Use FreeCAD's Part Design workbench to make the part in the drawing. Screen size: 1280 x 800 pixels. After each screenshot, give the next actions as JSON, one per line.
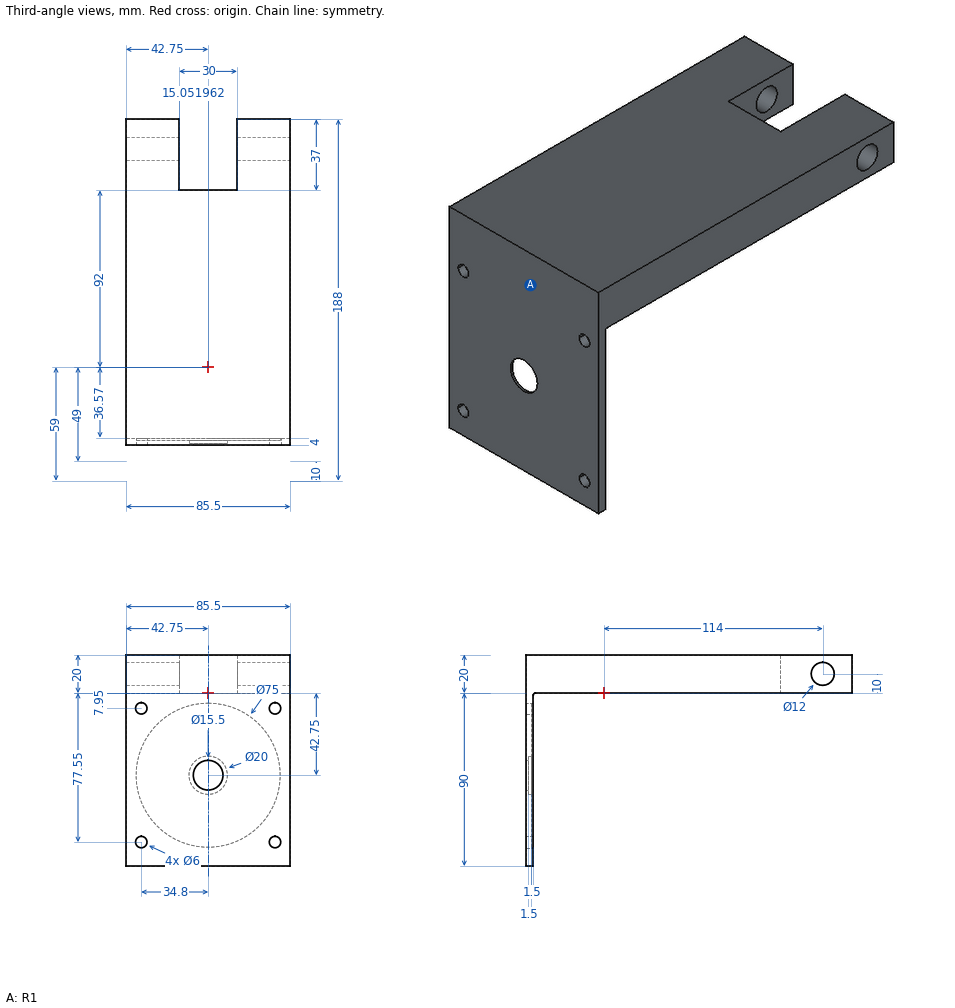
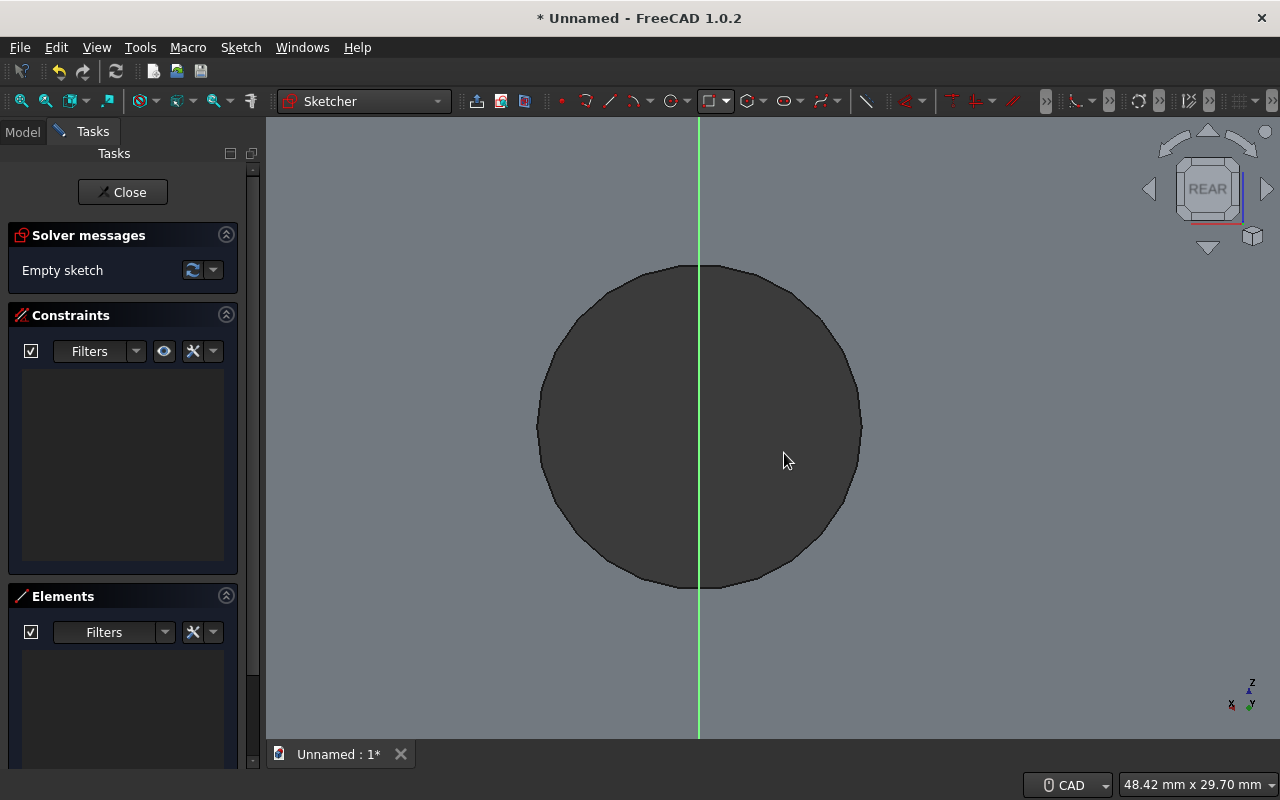
{"action": "key", "text": "g c"}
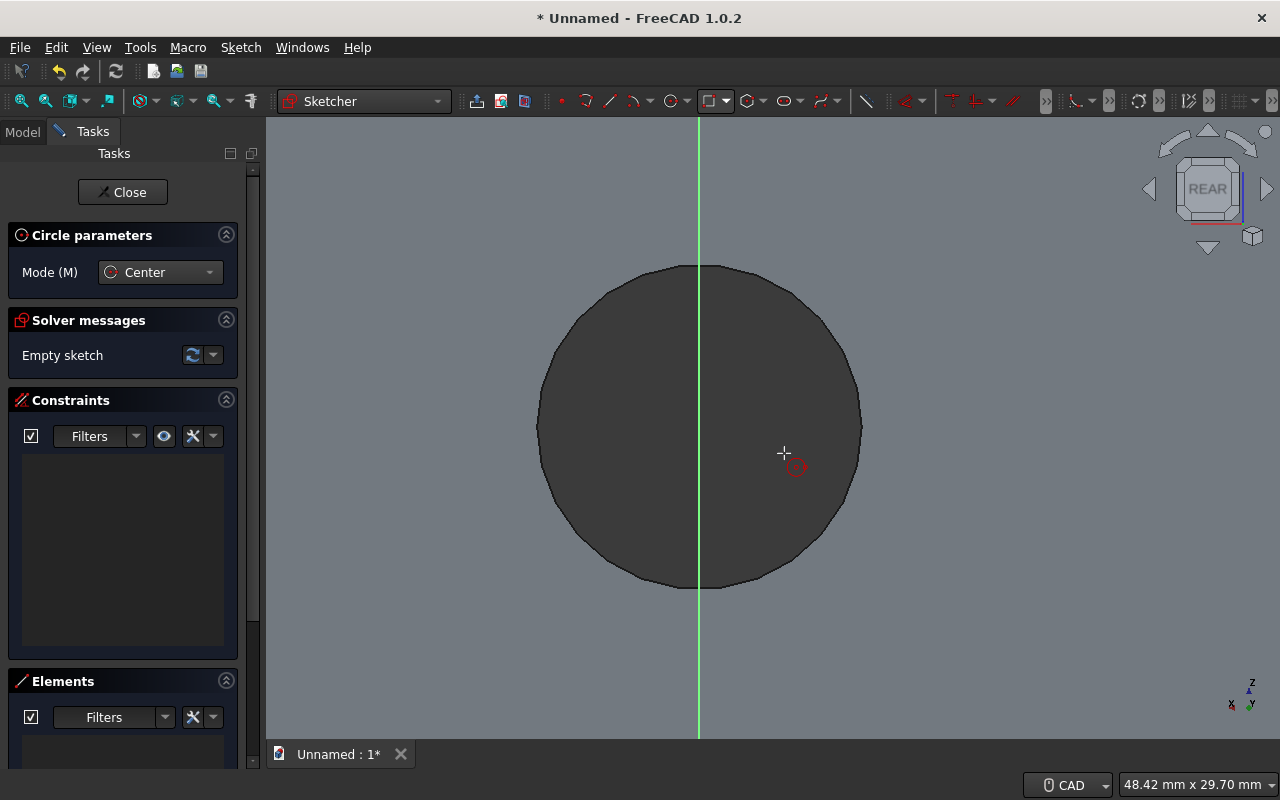
{"action": "left_click", "coordinate": [699, 427]}
{"action": "mouse_move", "coordinate": [848, 279]}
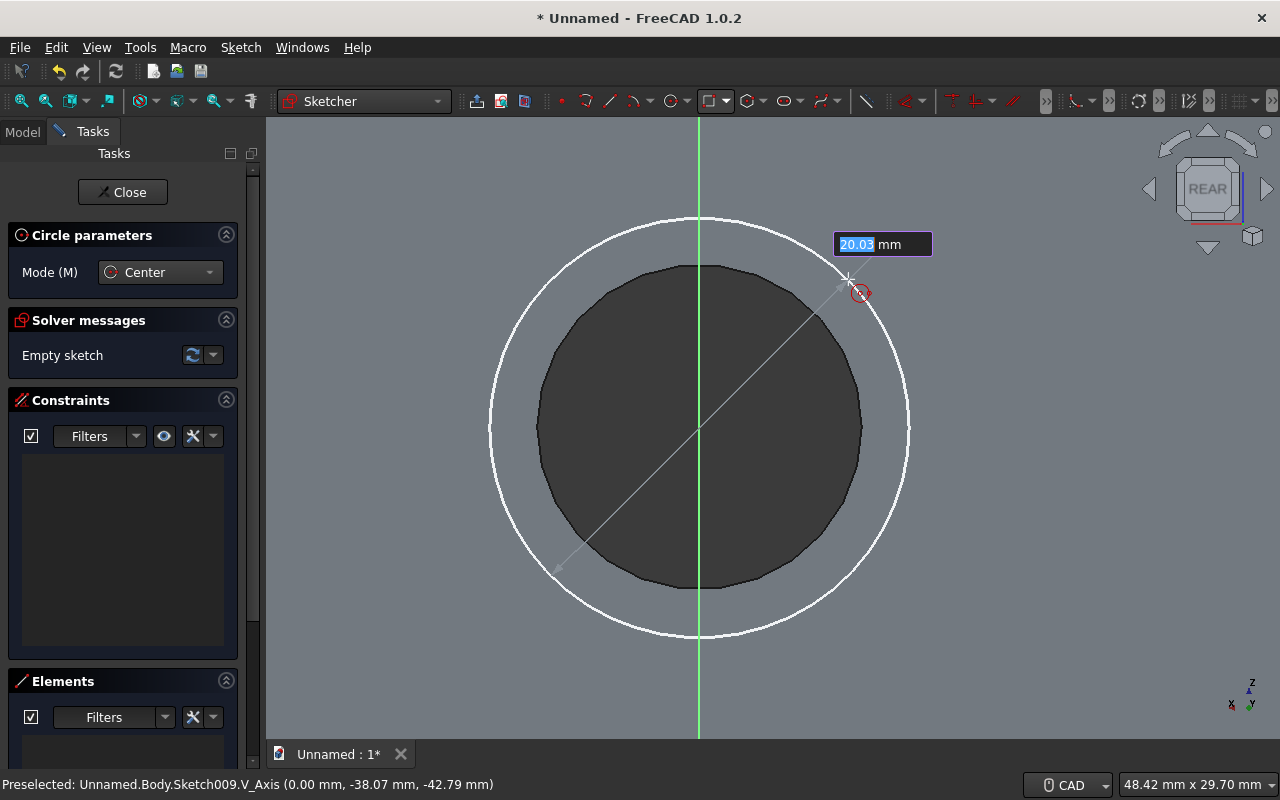
{"action": "type", "text": "20"}
{"action": "key", "text": "Return"}
{"action": "key", "text": "Escape"}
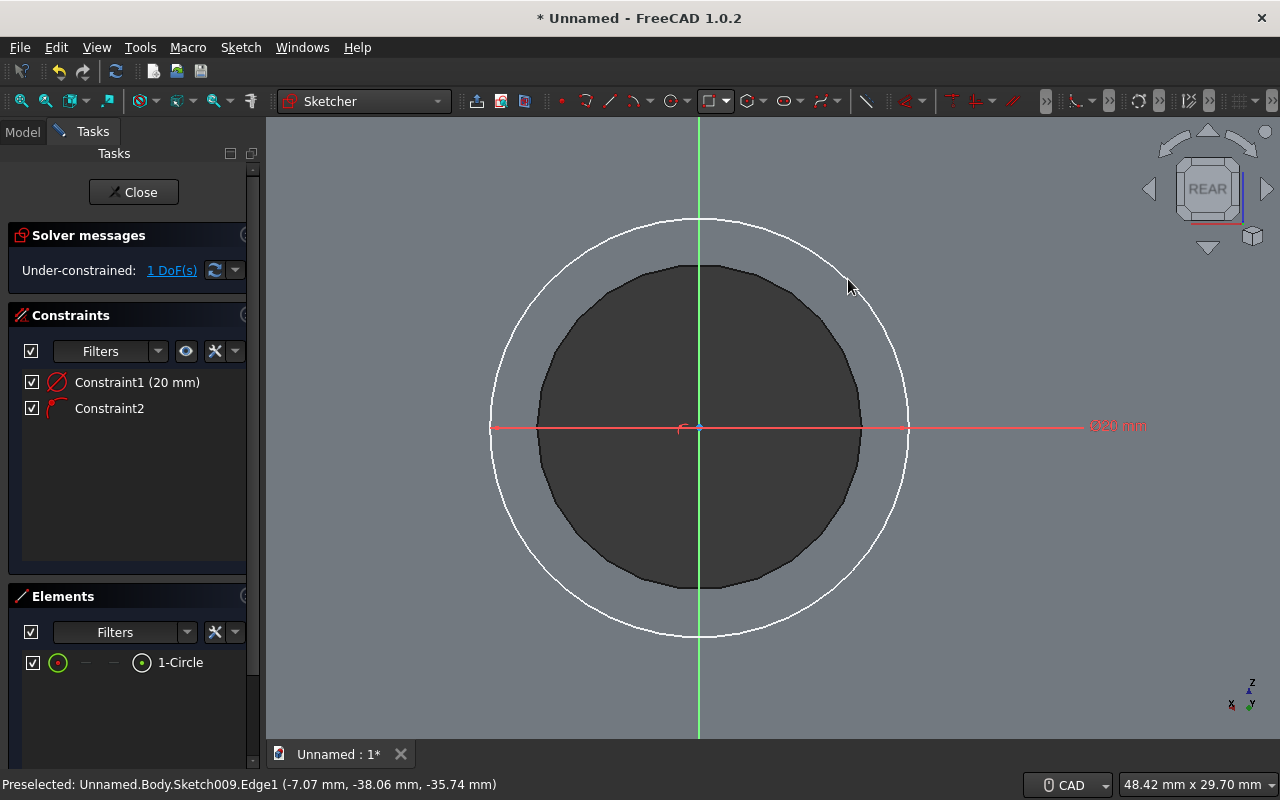
{"action": "key", "text": "d"}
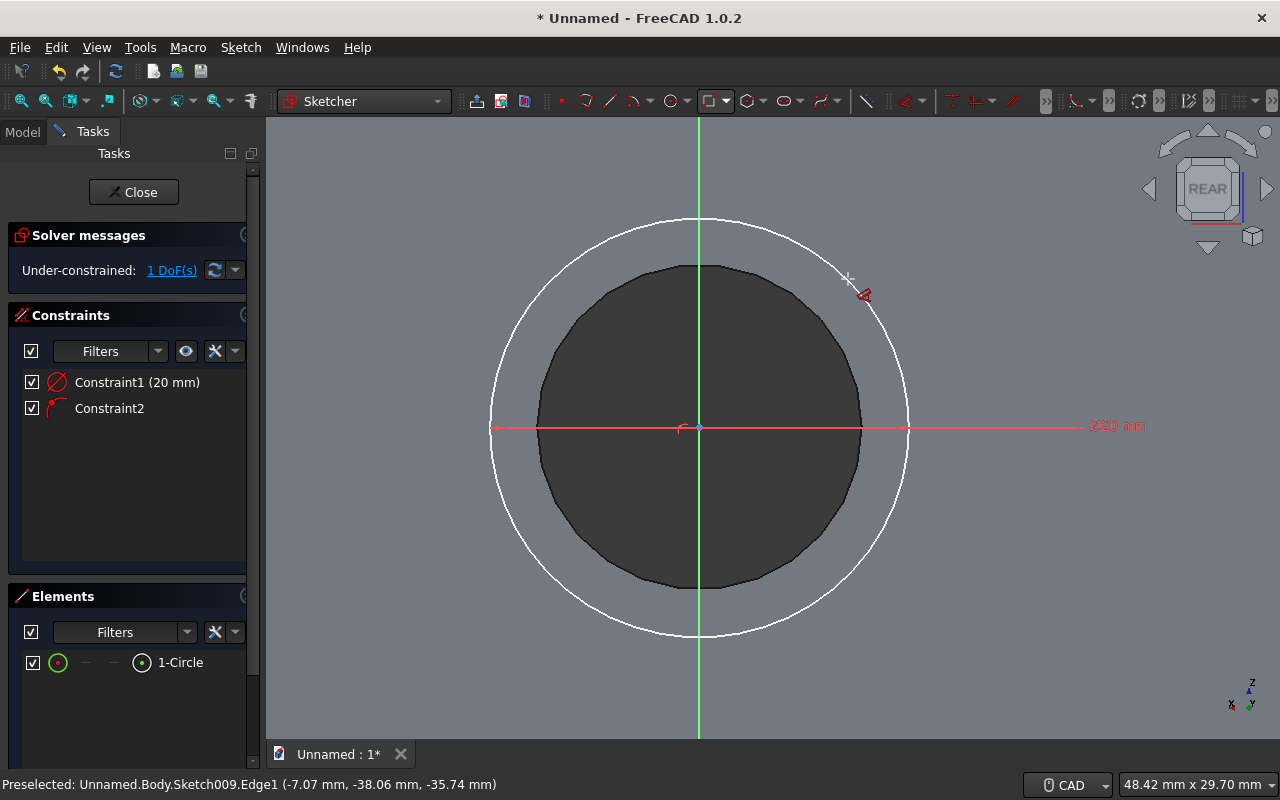
{"action": "left_click", "coordinate": [699, 428]}
{"action": "left_click", "coordinate": [733, 287]}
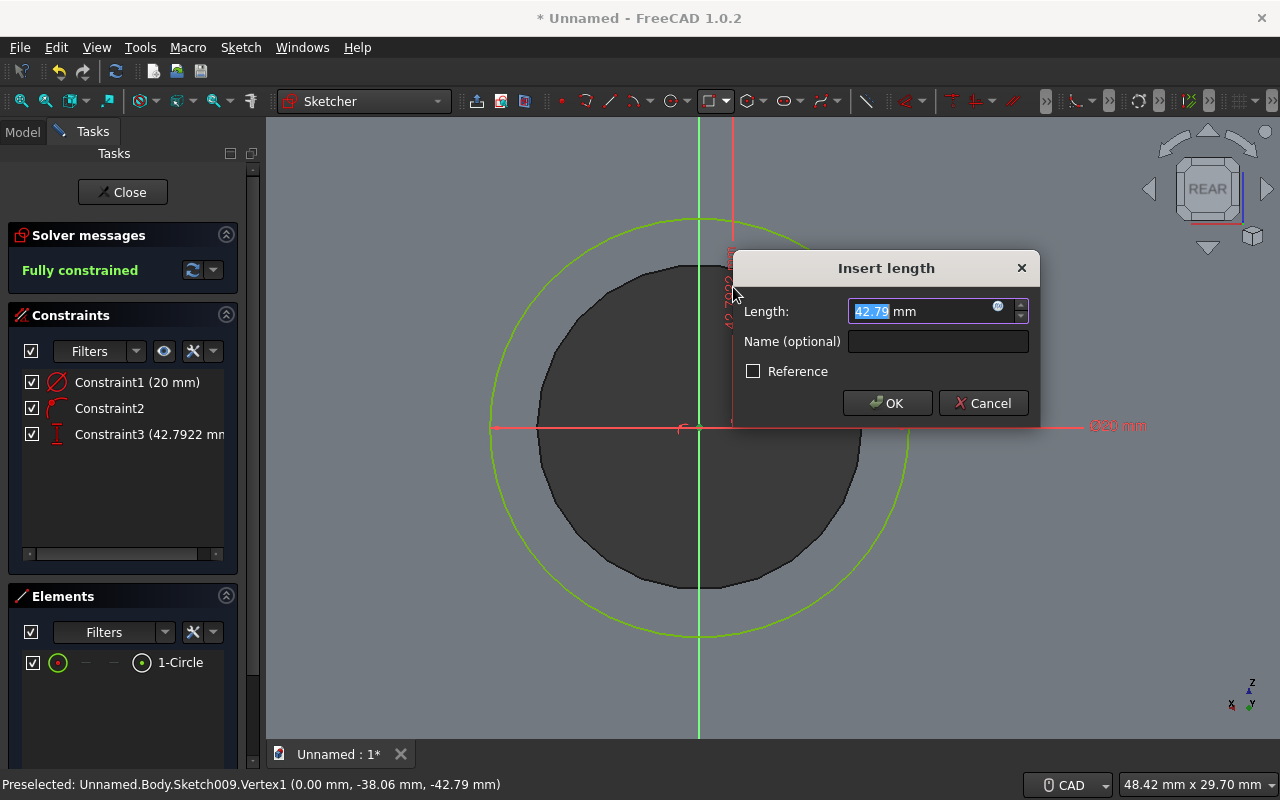
{"action": "type", "text": "42.75"}
{"action": "key", "text": "Return"}
{"action": "key", "text": "Escape"}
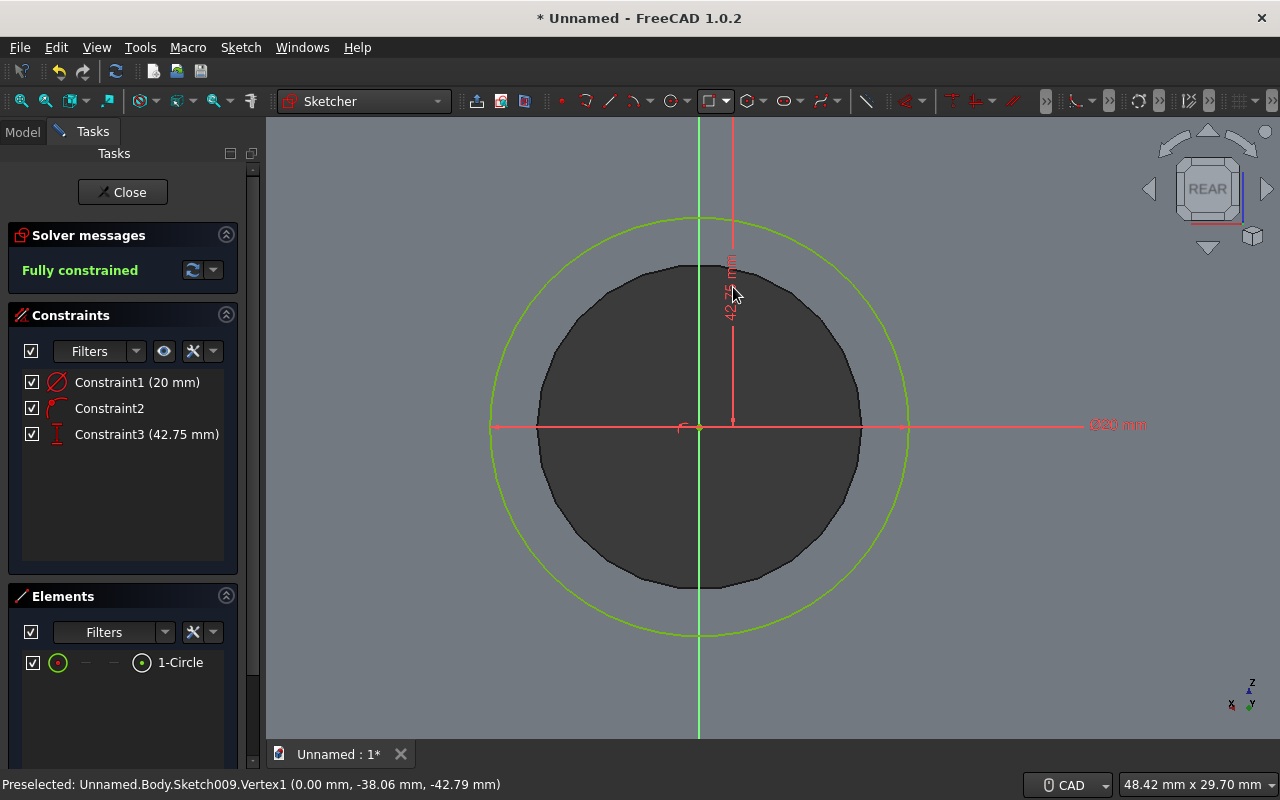
{"action": "left_click", "coordinate": [123, 192]}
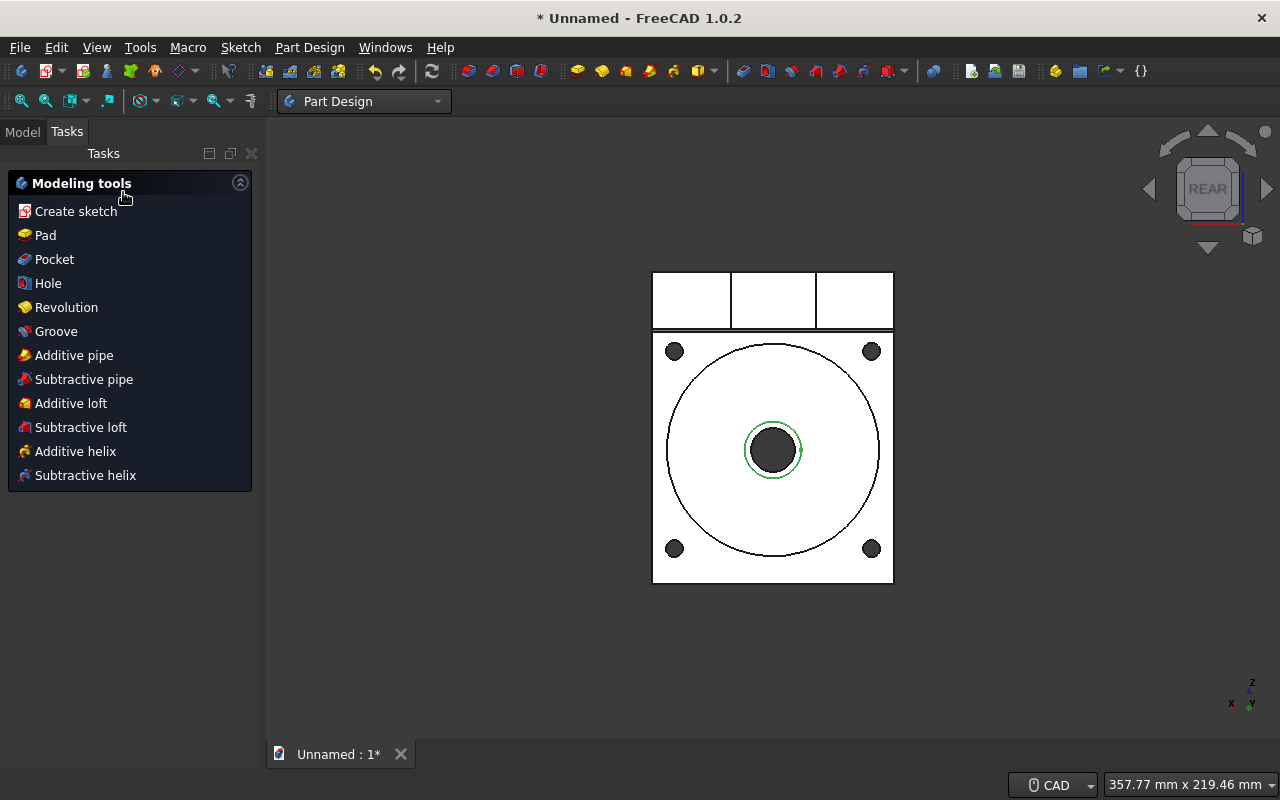
{"action": "left_click", "coordinate": [744, 72]}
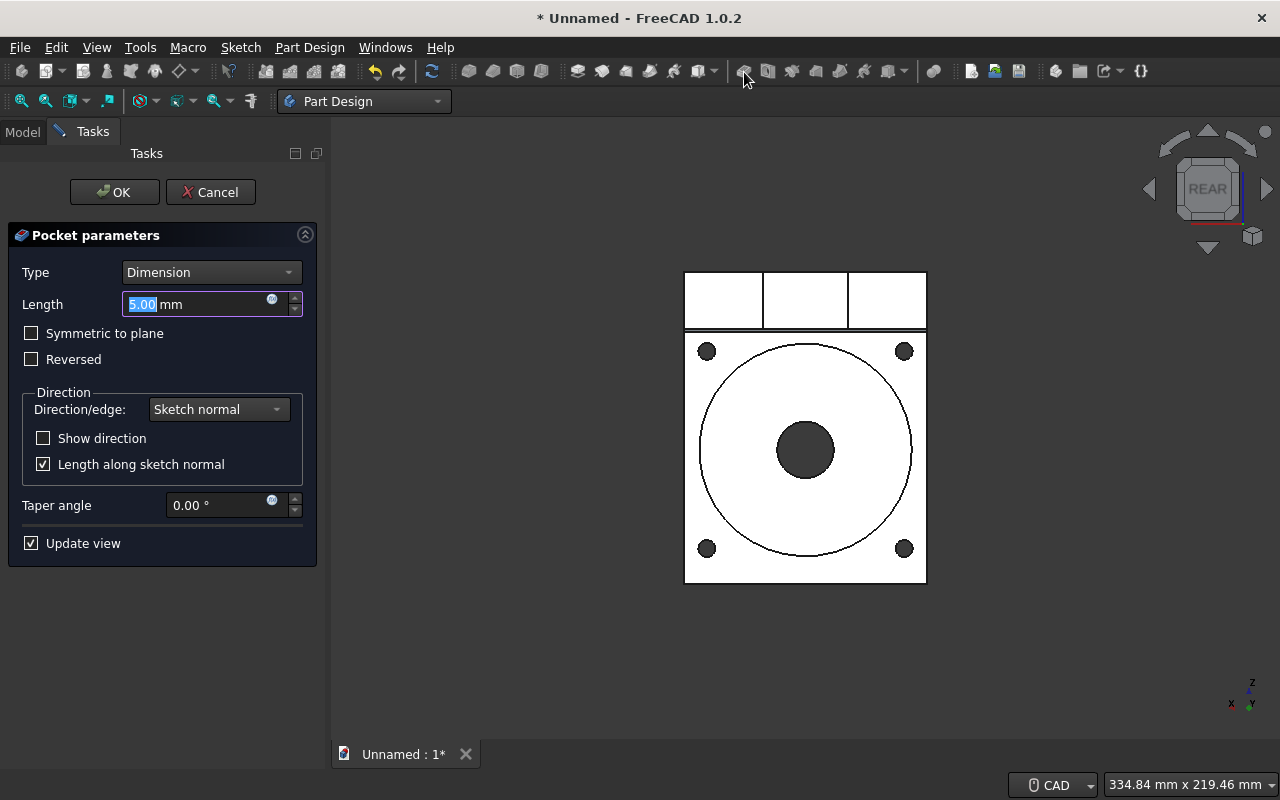
{"action": "type", "text": "1.5"}
{"action": "key", "text": "Tab"}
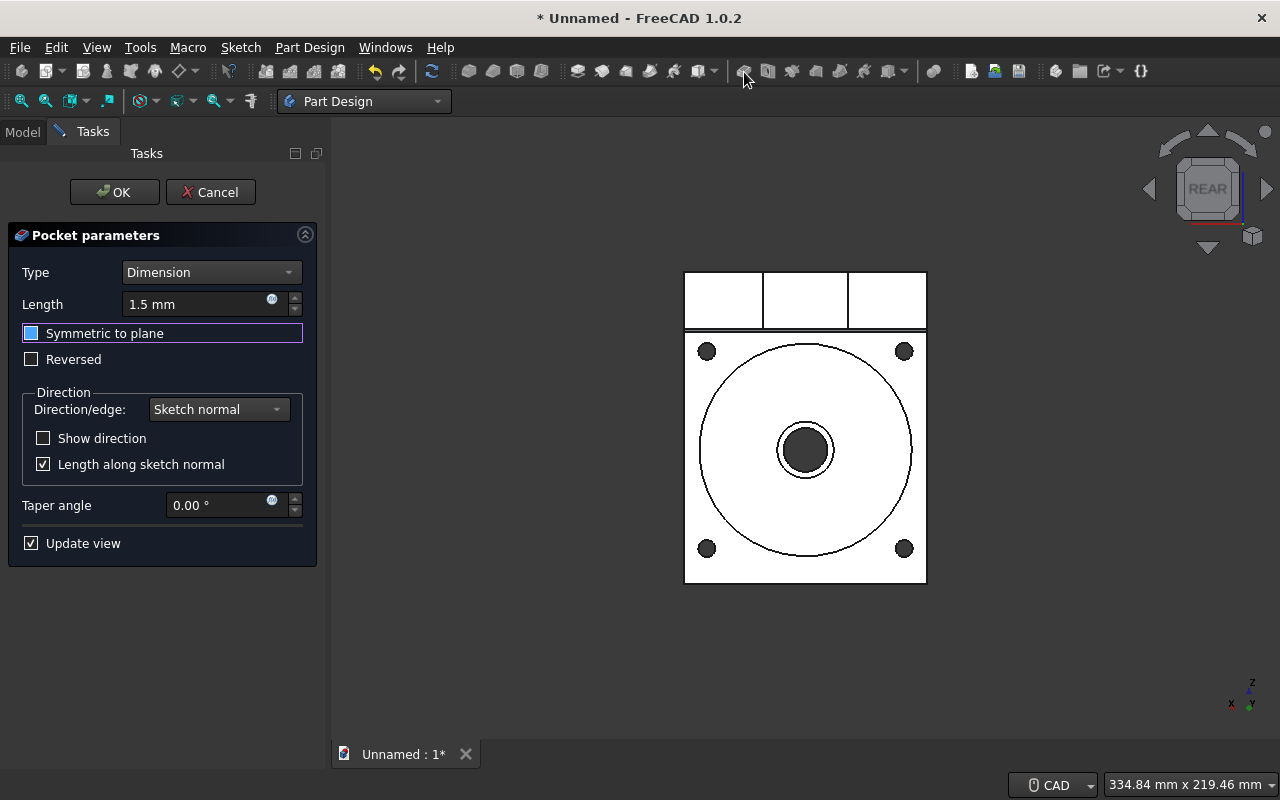
{"action": "left_click", "coordinate": [115, 192]}